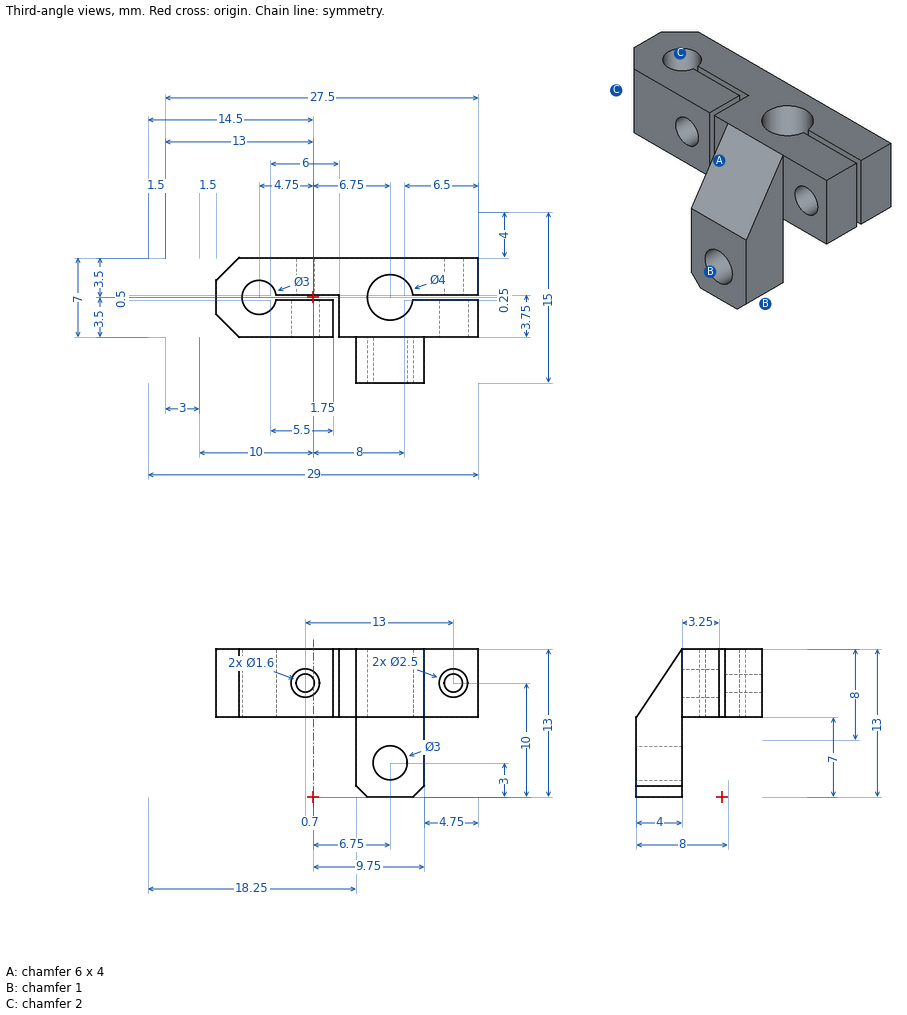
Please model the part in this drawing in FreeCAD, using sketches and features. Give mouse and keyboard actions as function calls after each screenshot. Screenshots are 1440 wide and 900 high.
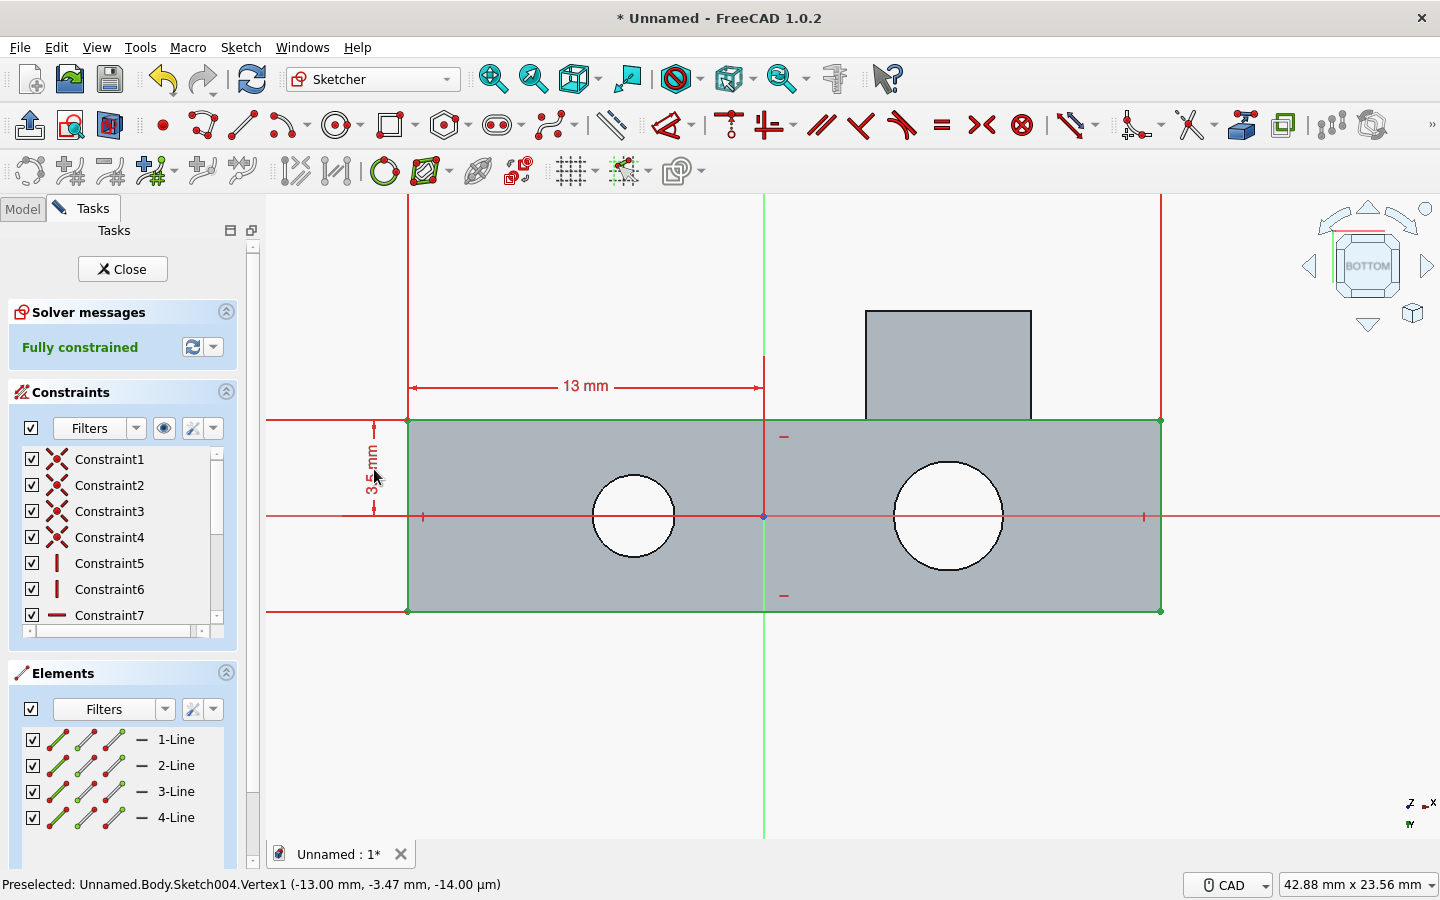
click(123, 269)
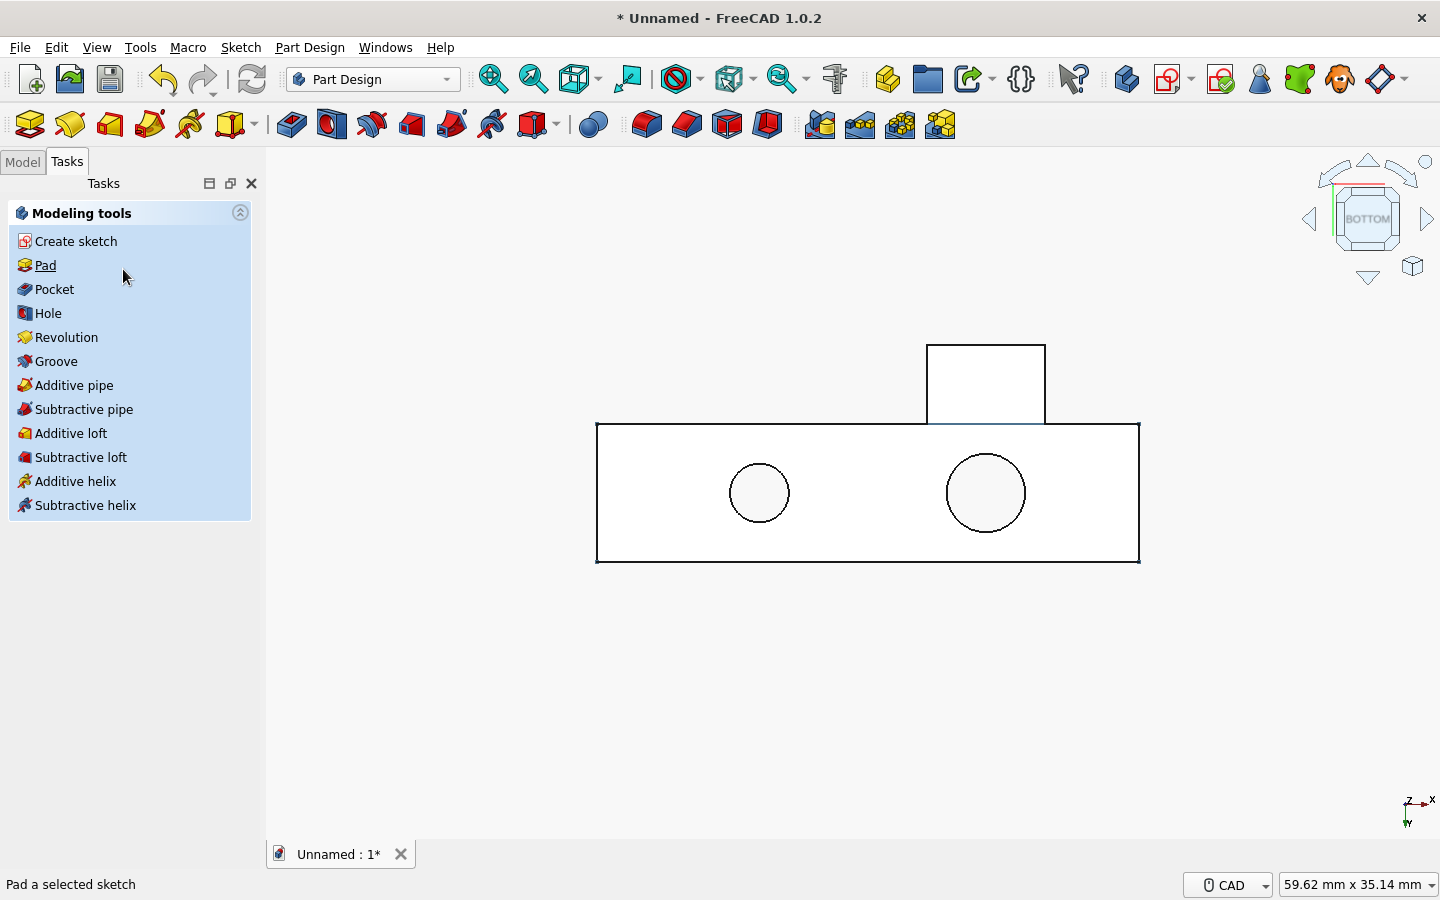
click(292, 124)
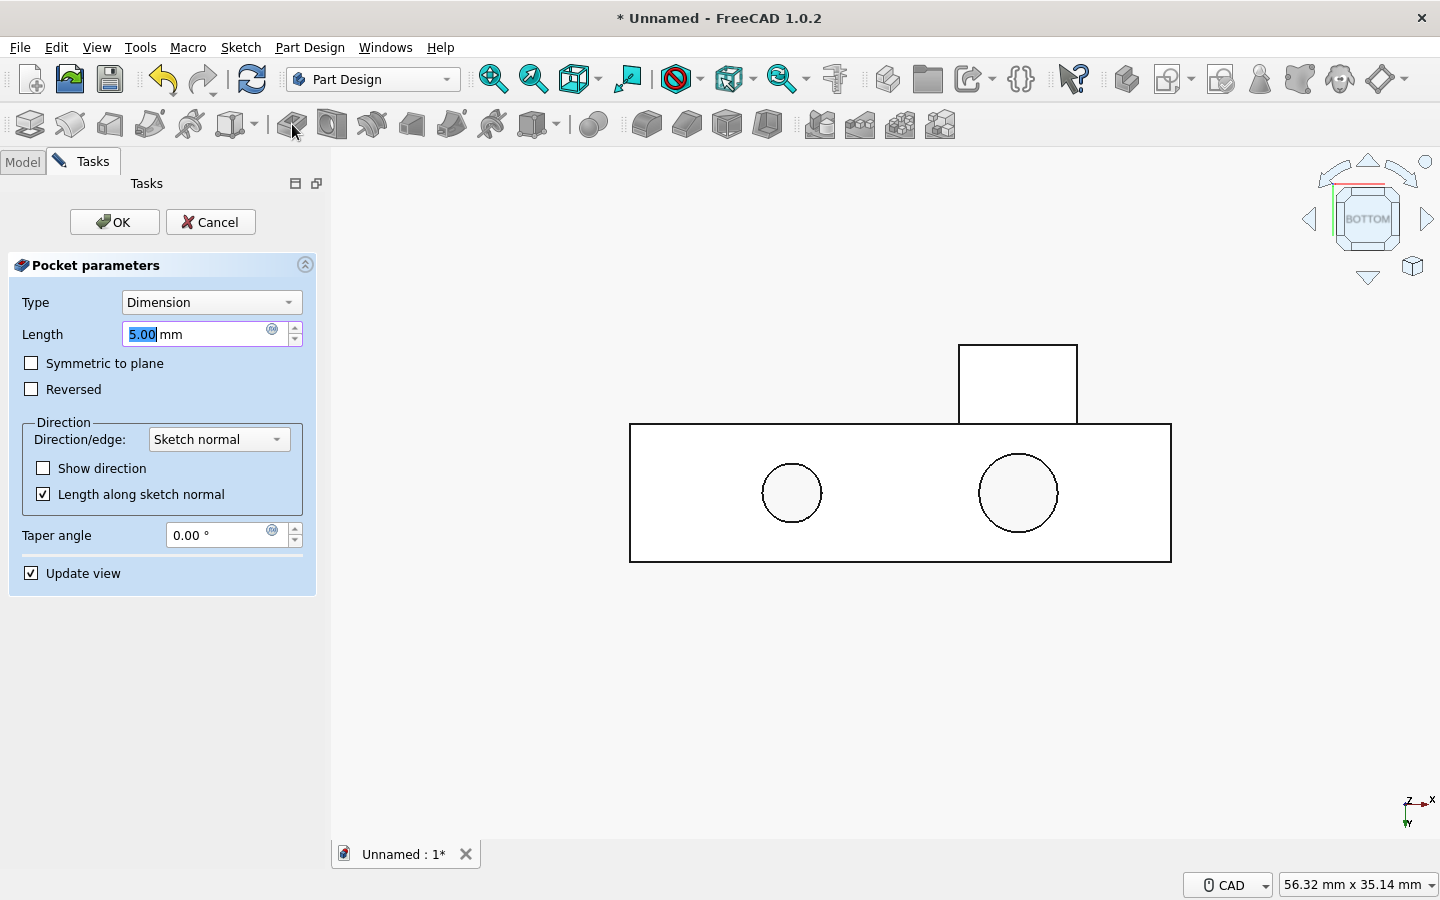
text(7)
key(Tab)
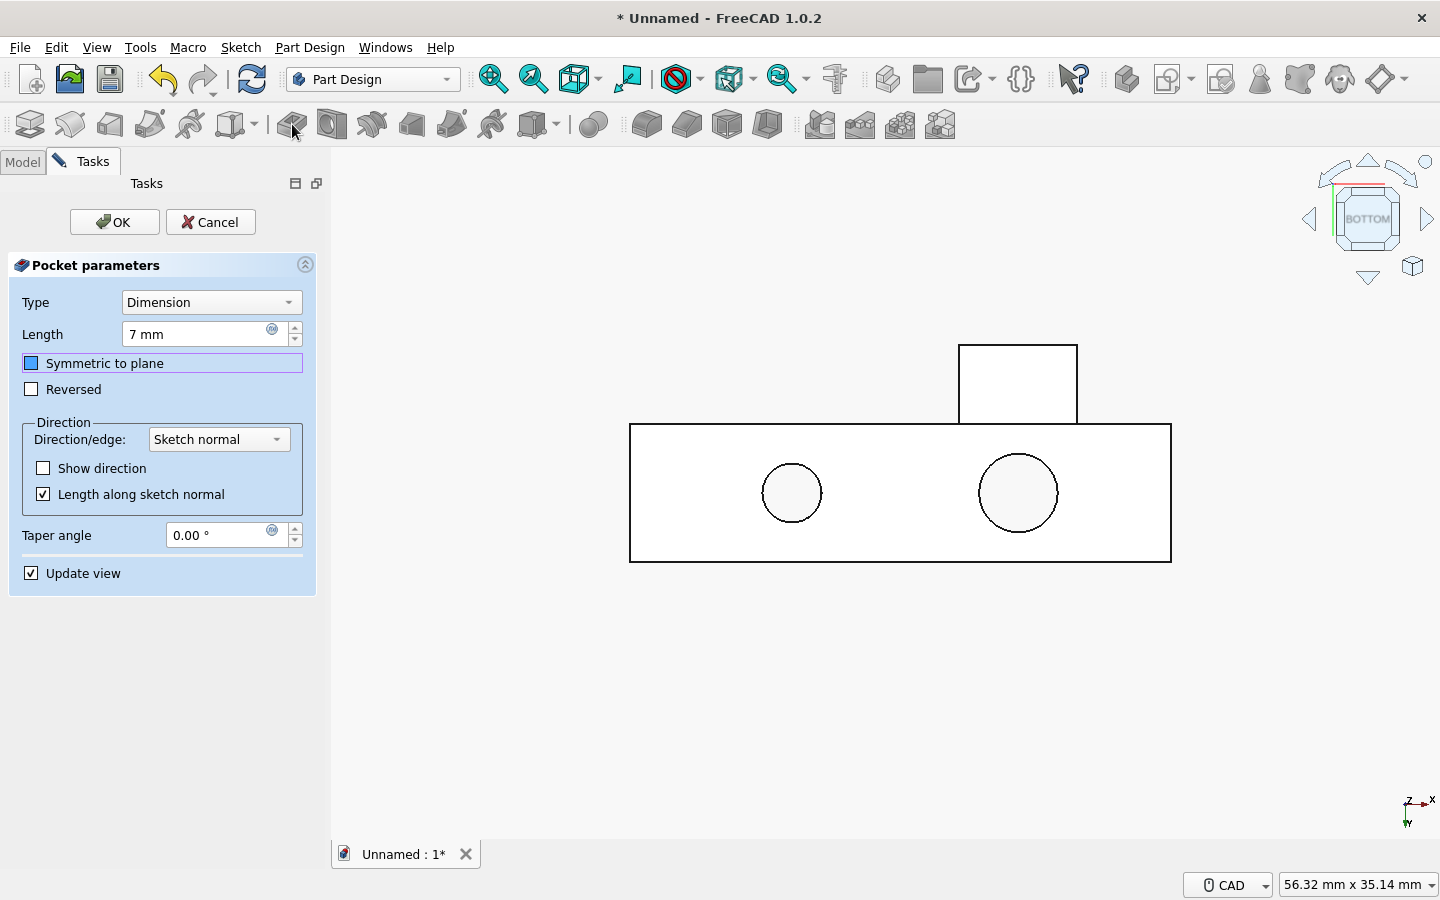
click(115, 222)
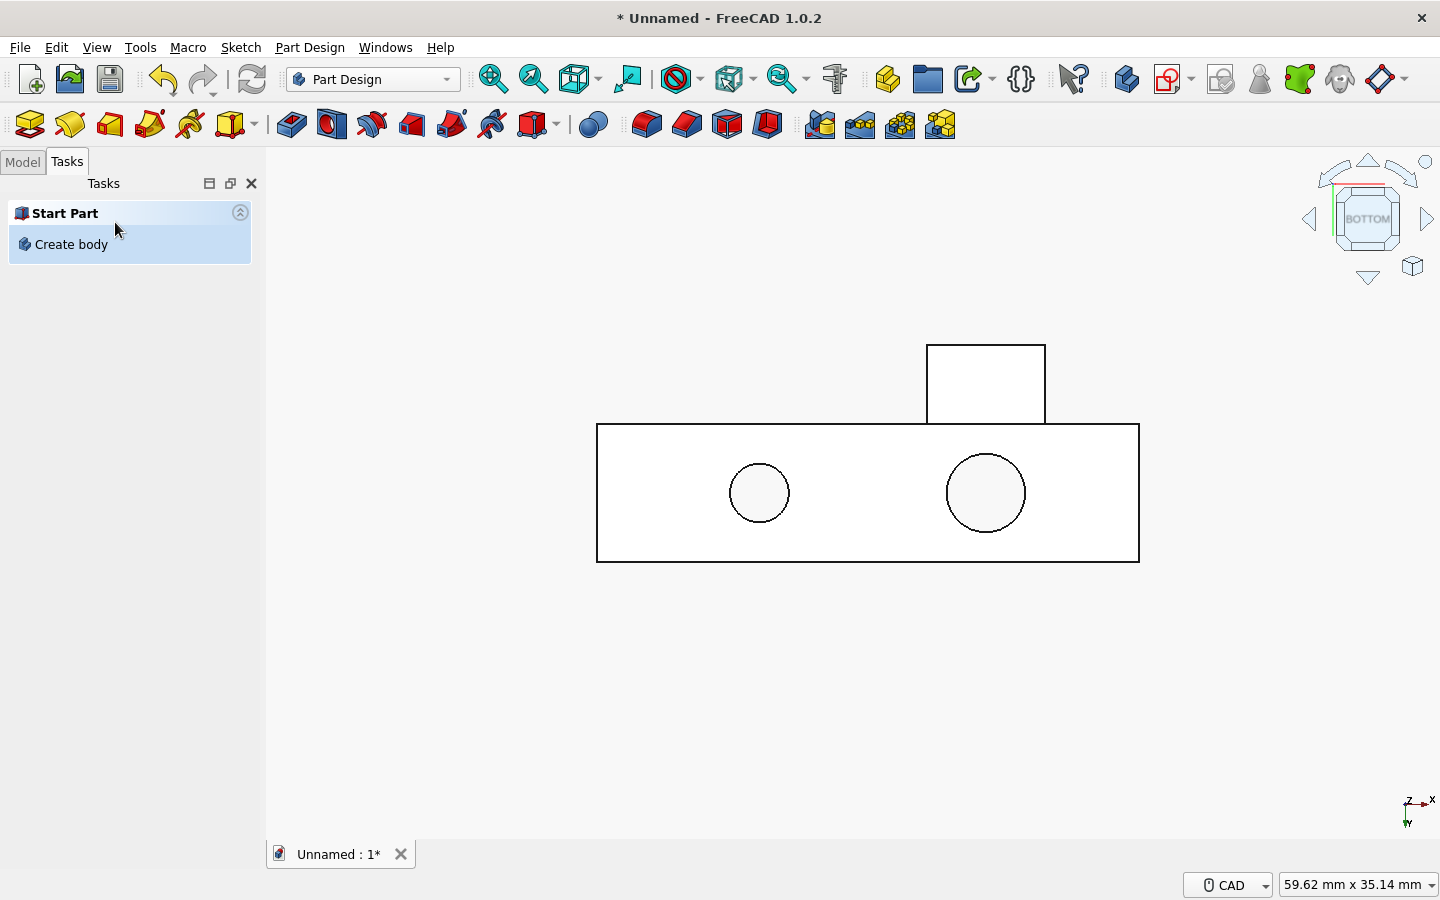
key(0)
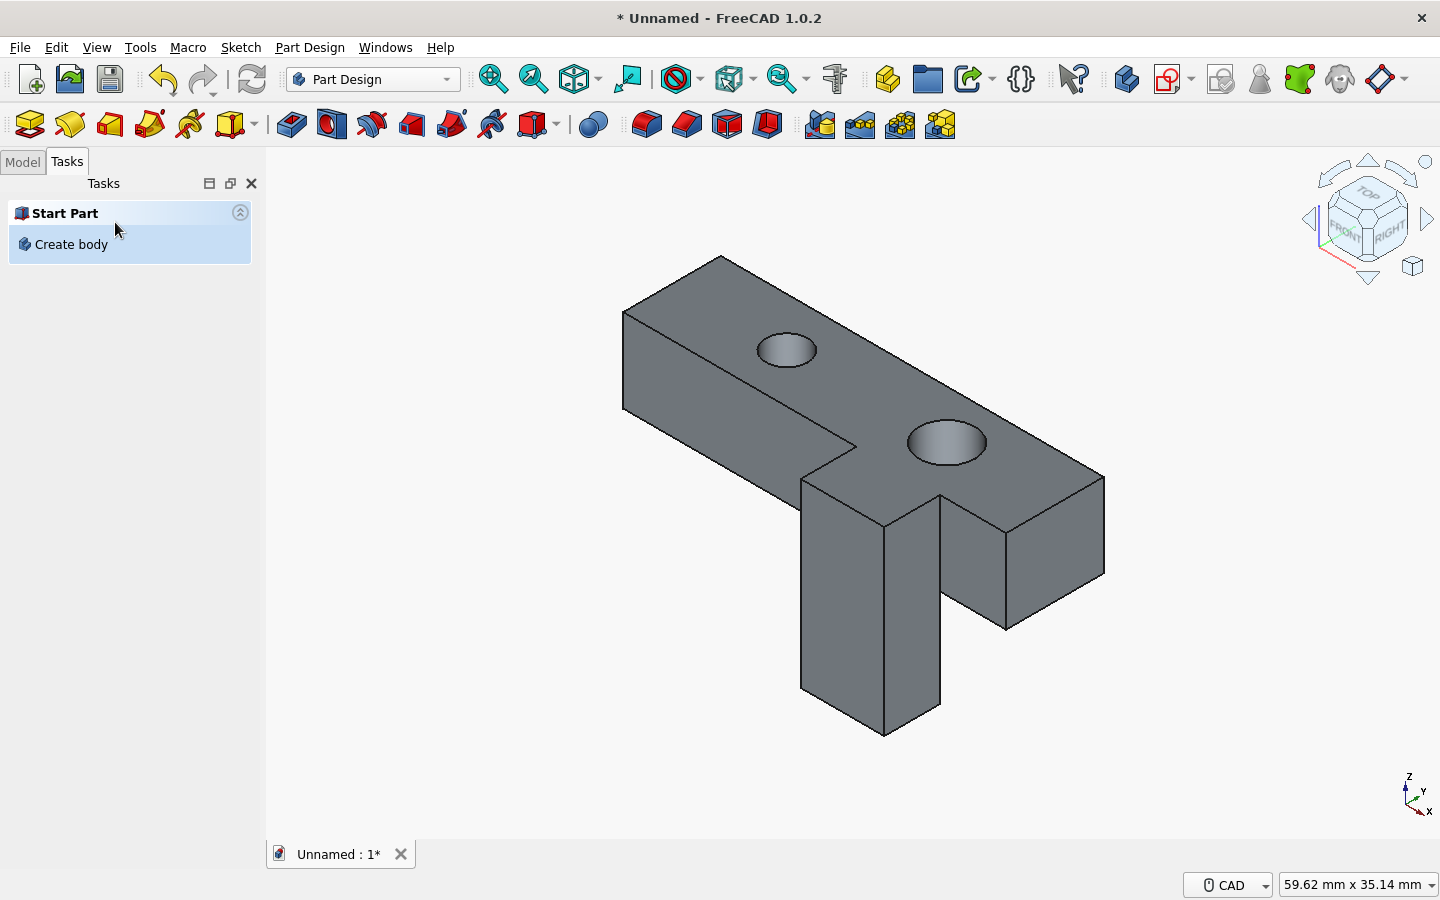
click(843, 502)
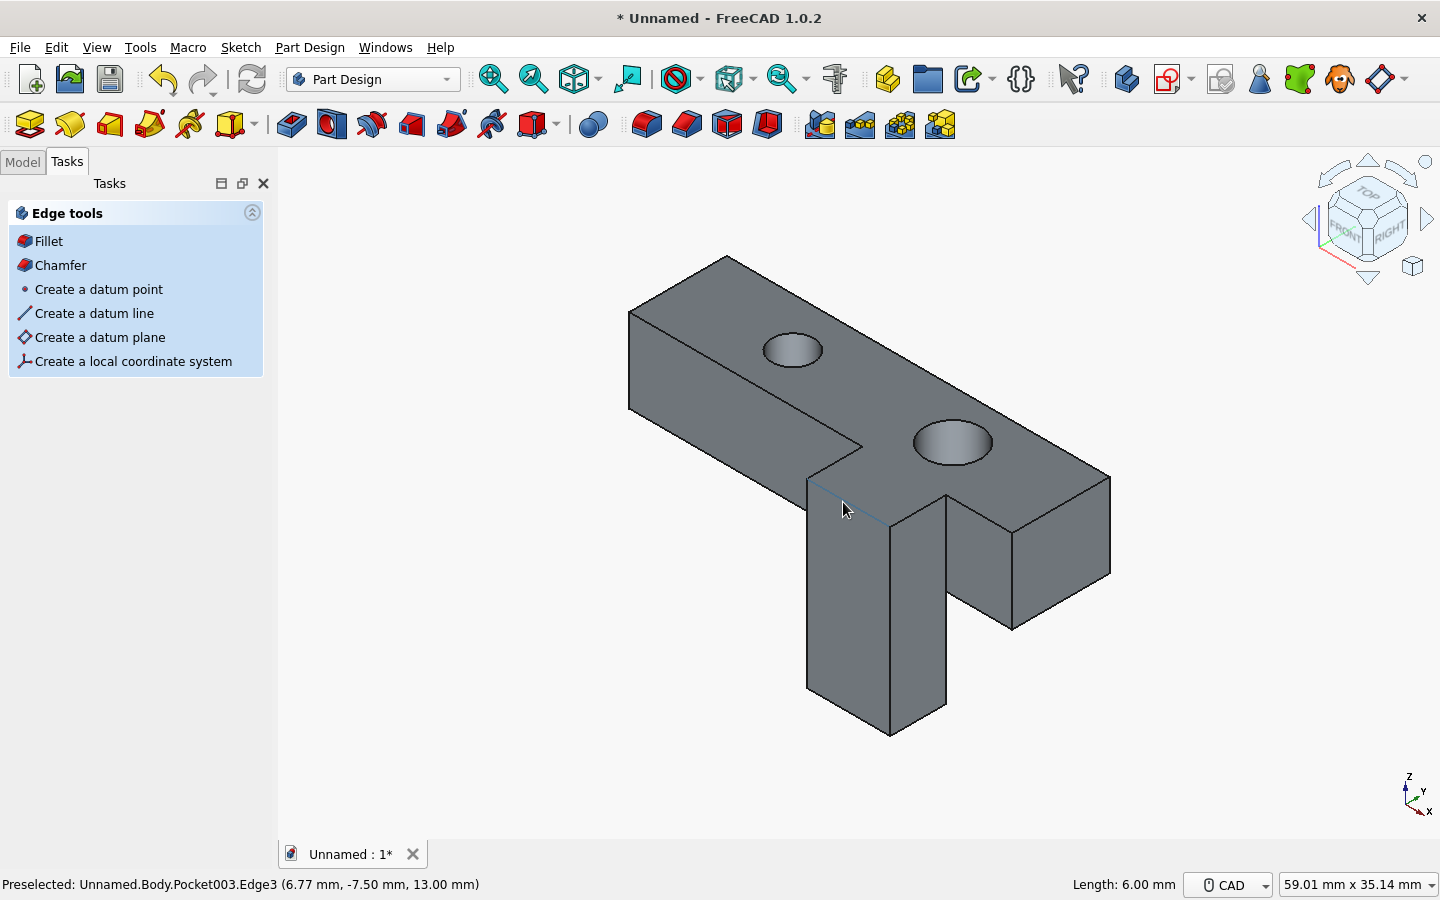
click(688, 124)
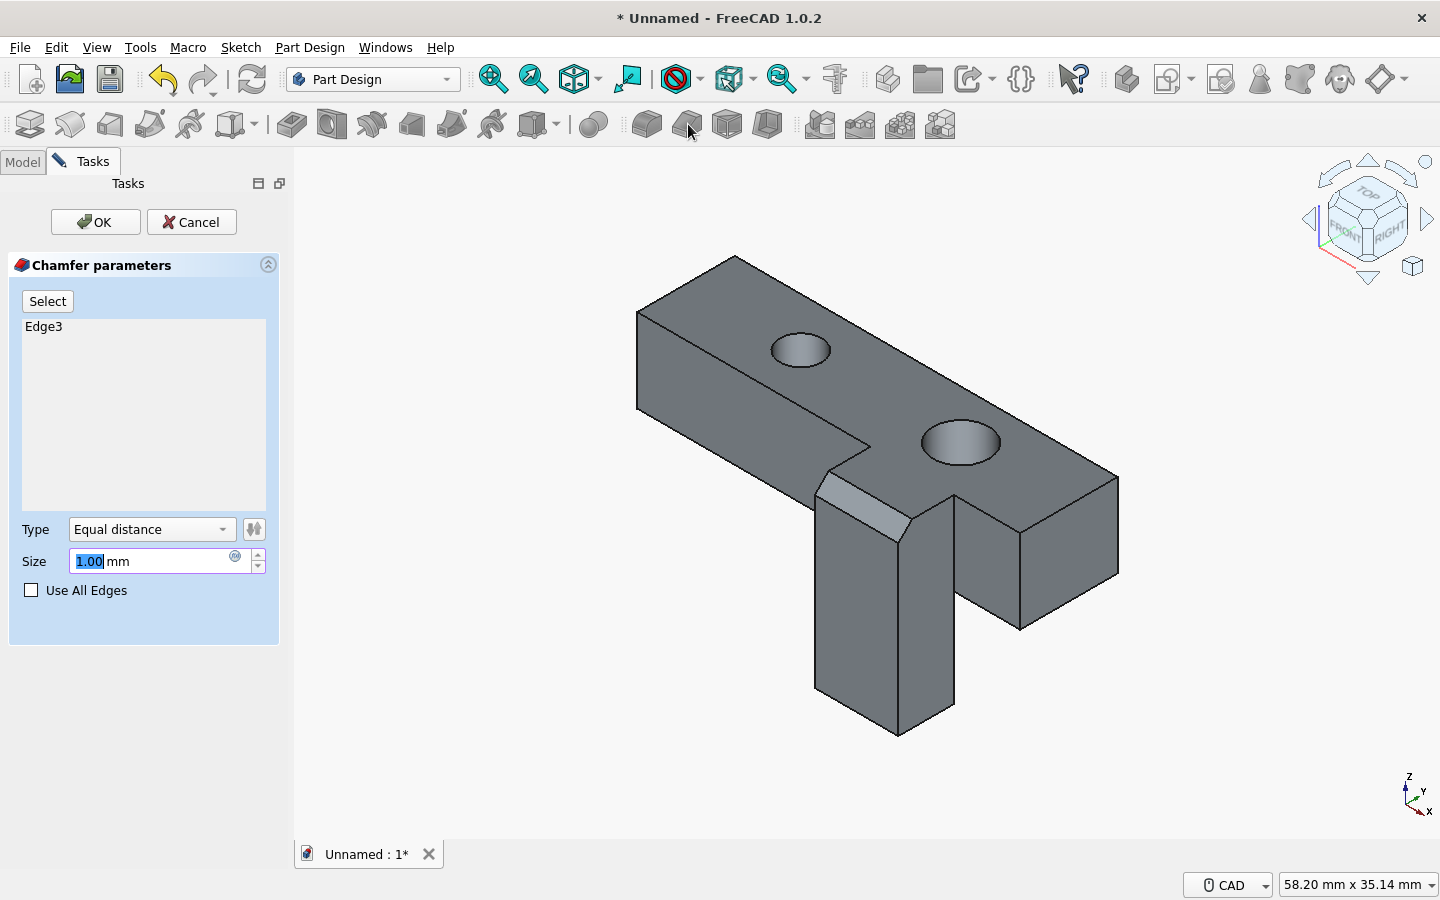
text(6)
key(Tab)